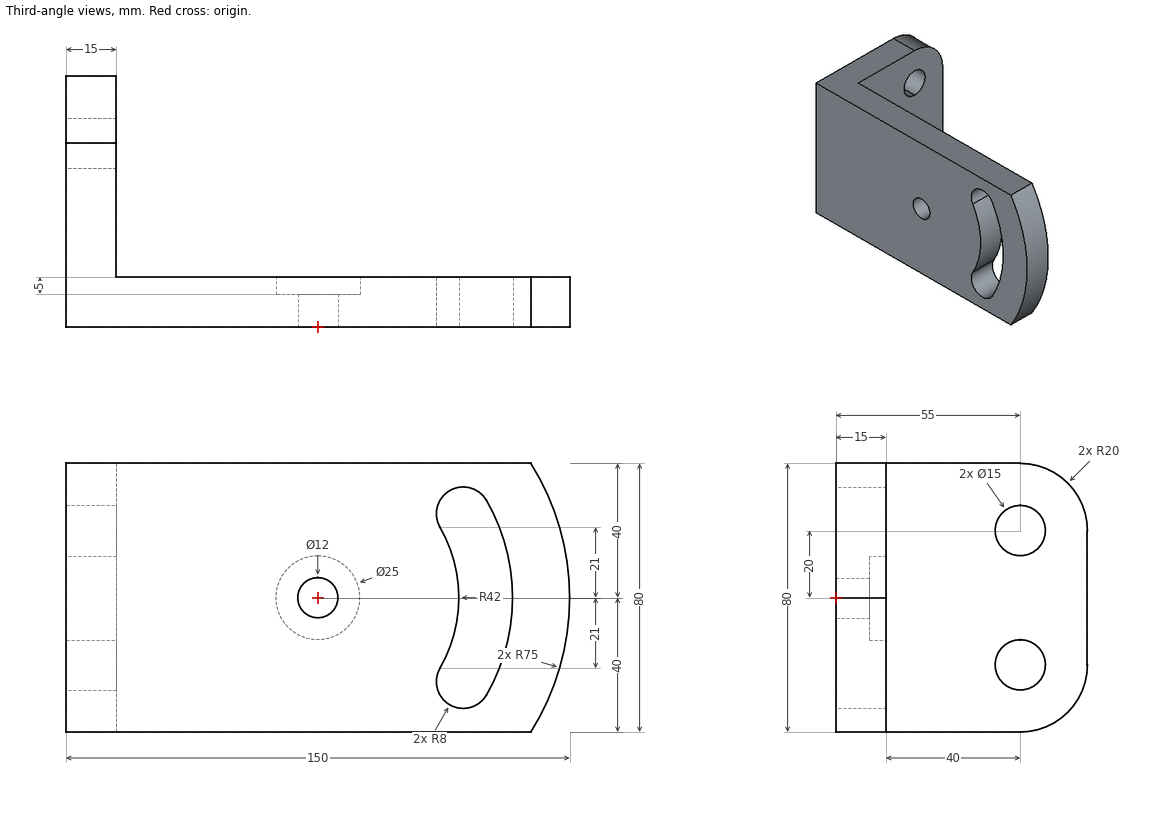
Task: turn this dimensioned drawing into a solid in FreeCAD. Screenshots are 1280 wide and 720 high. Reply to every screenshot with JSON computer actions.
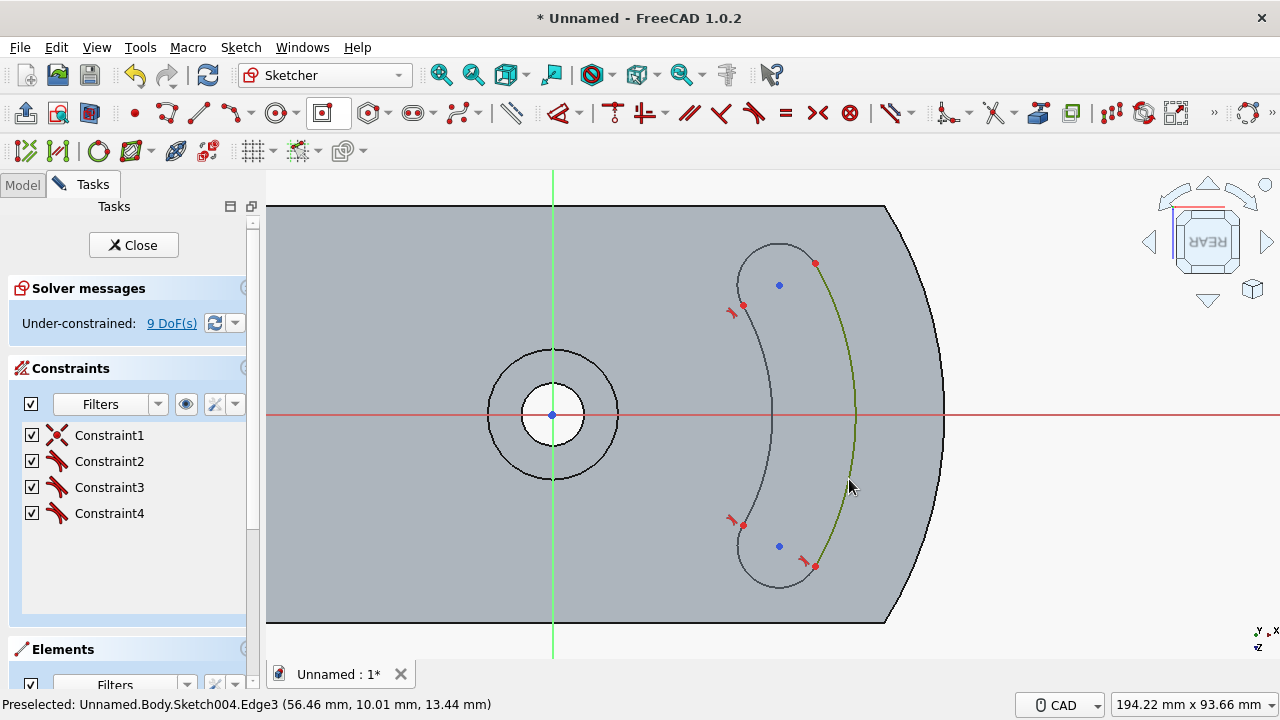
{"action": "left_click", "coordinate": [783, 244]}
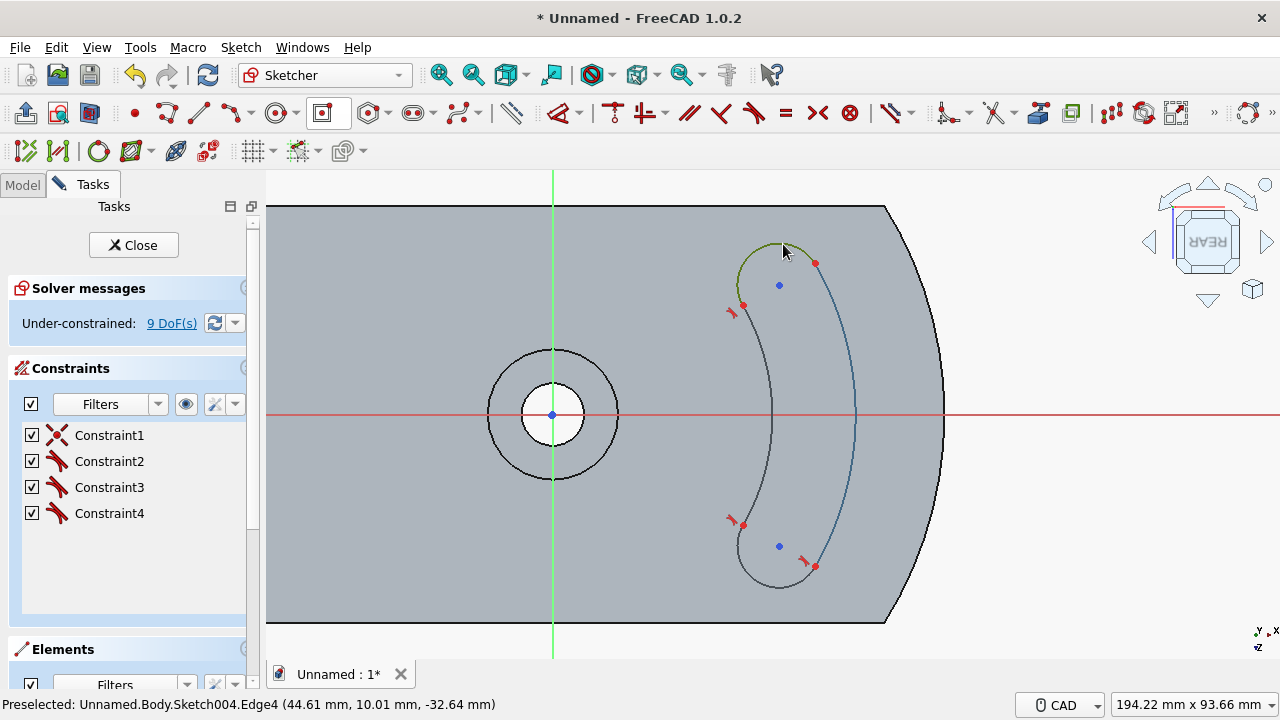
{"action": "left_click", "coordinate": [754, 114]}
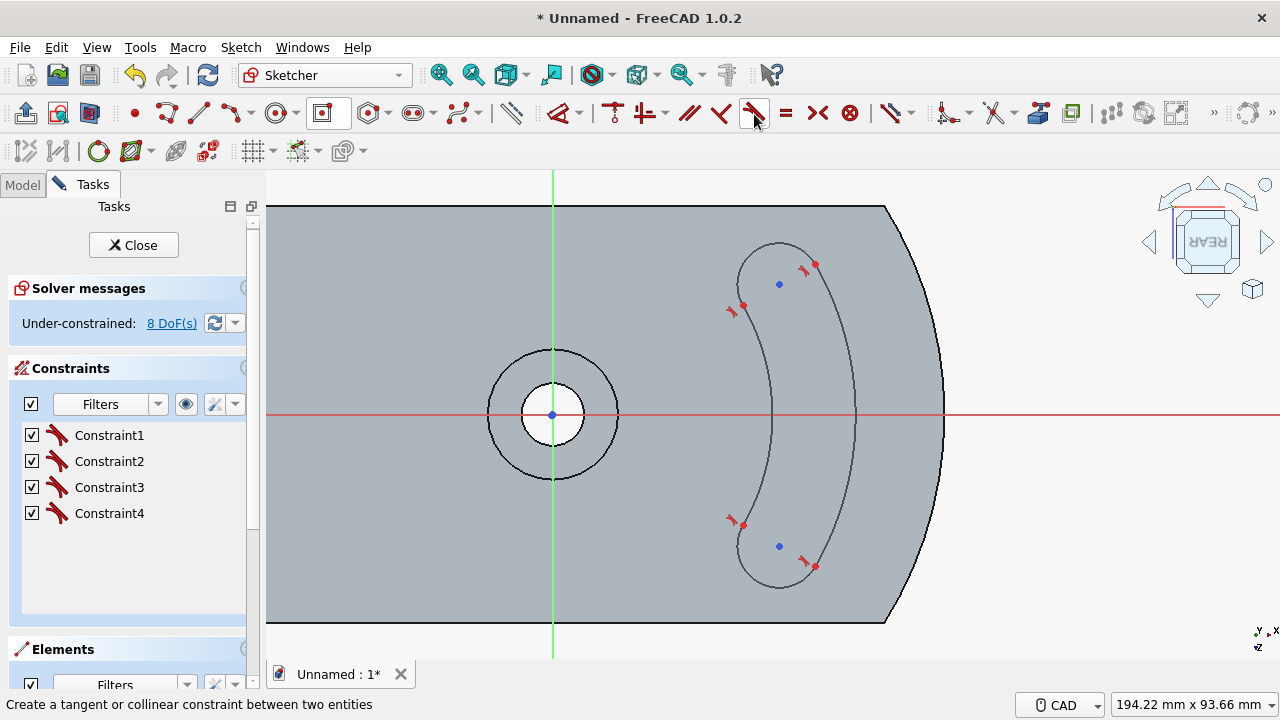
{"action": "left_click", "coordinate": [768, 461]}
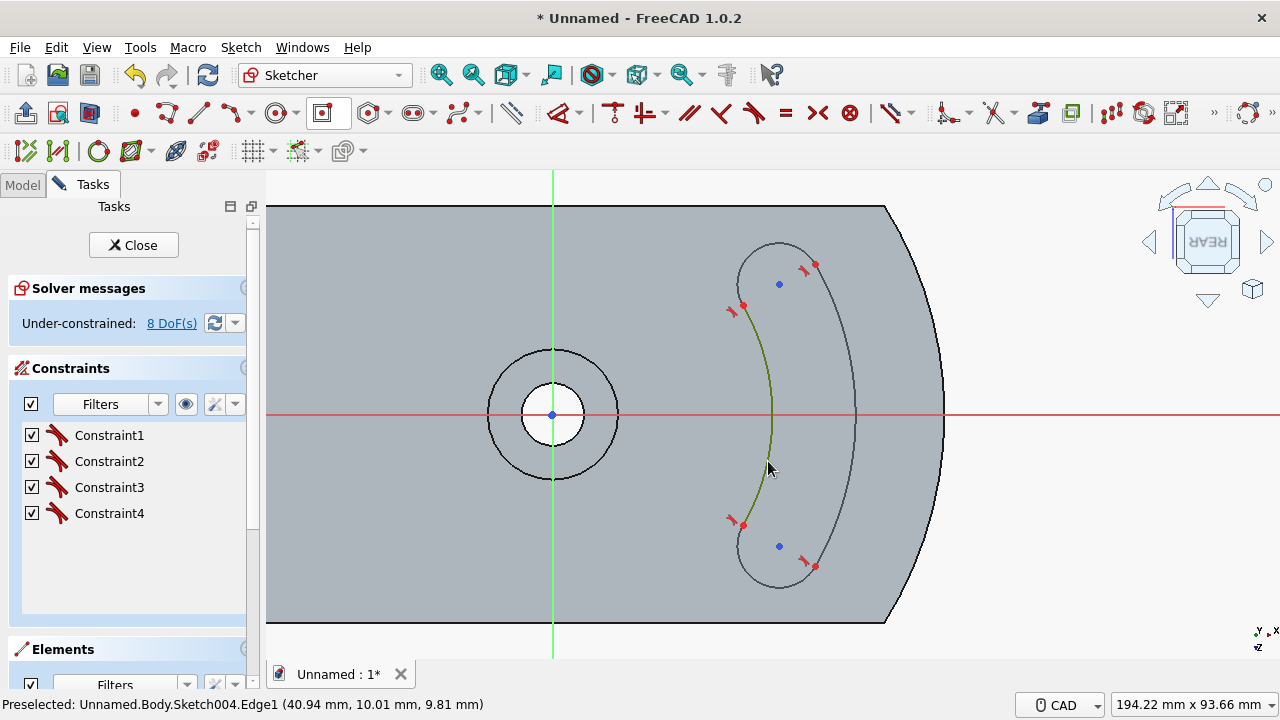
{"action": "left_click", "coordinate": [849, 479]}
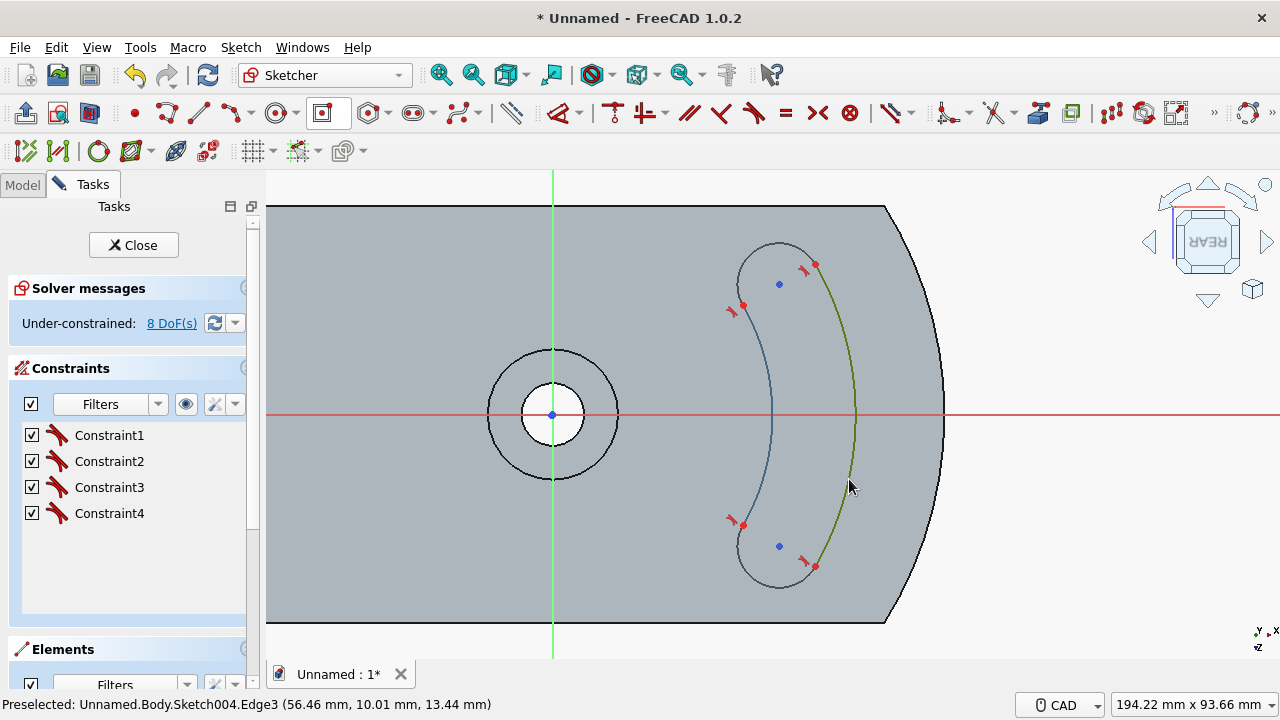
{"action": "left_click", "coordinate": [614, 114]}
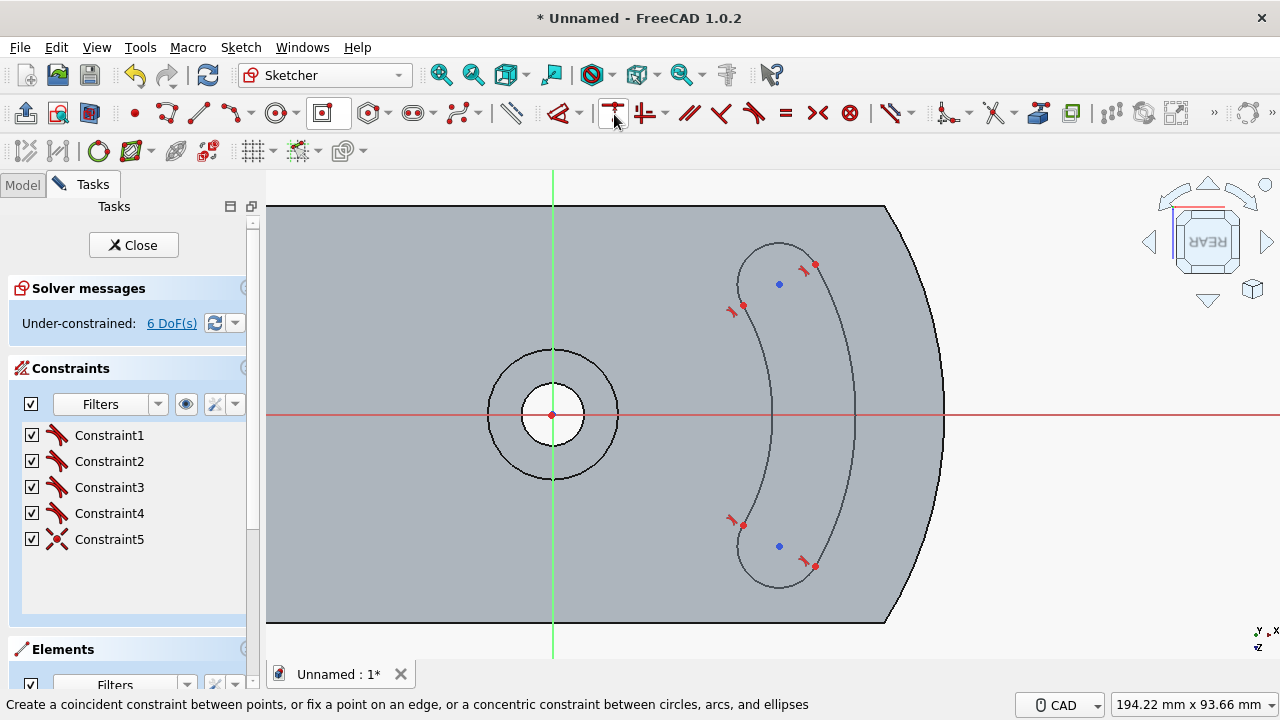
{"action": "left_click_drag", "start_coordinate": [542, 404], "coordinate": [563, 425]}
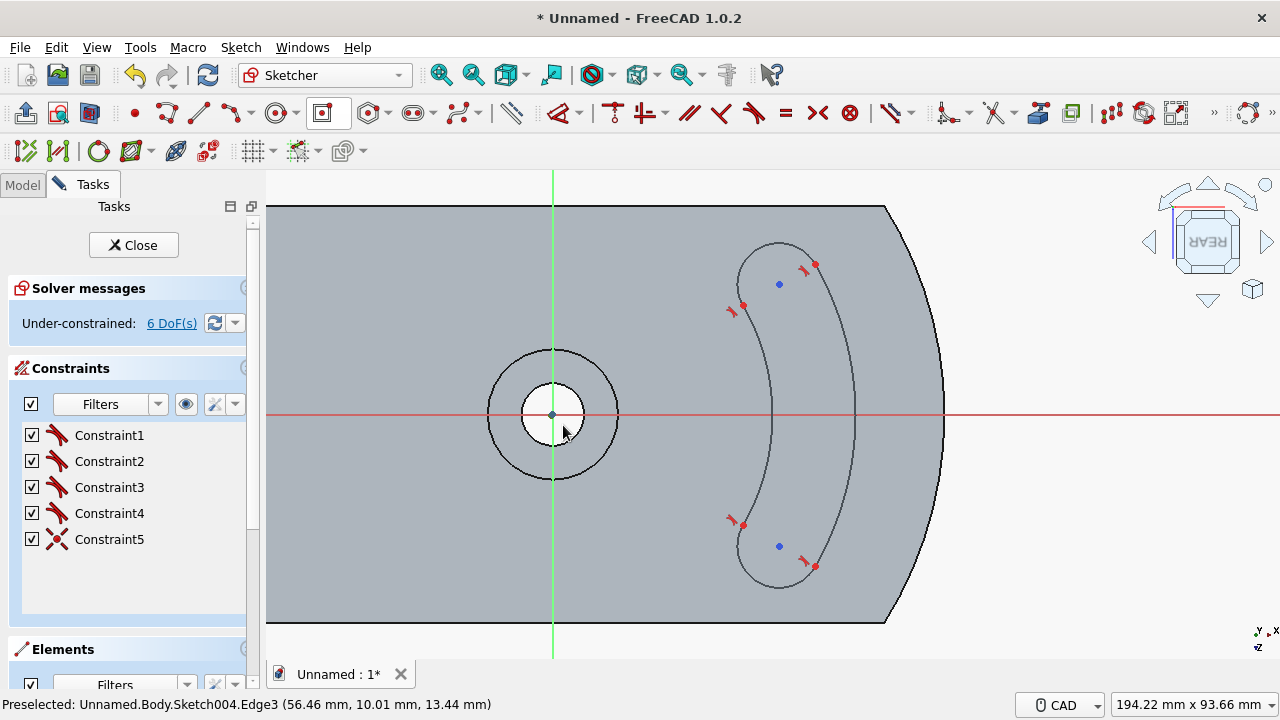
{"action": "left_click", "coordinate": [614, 114]}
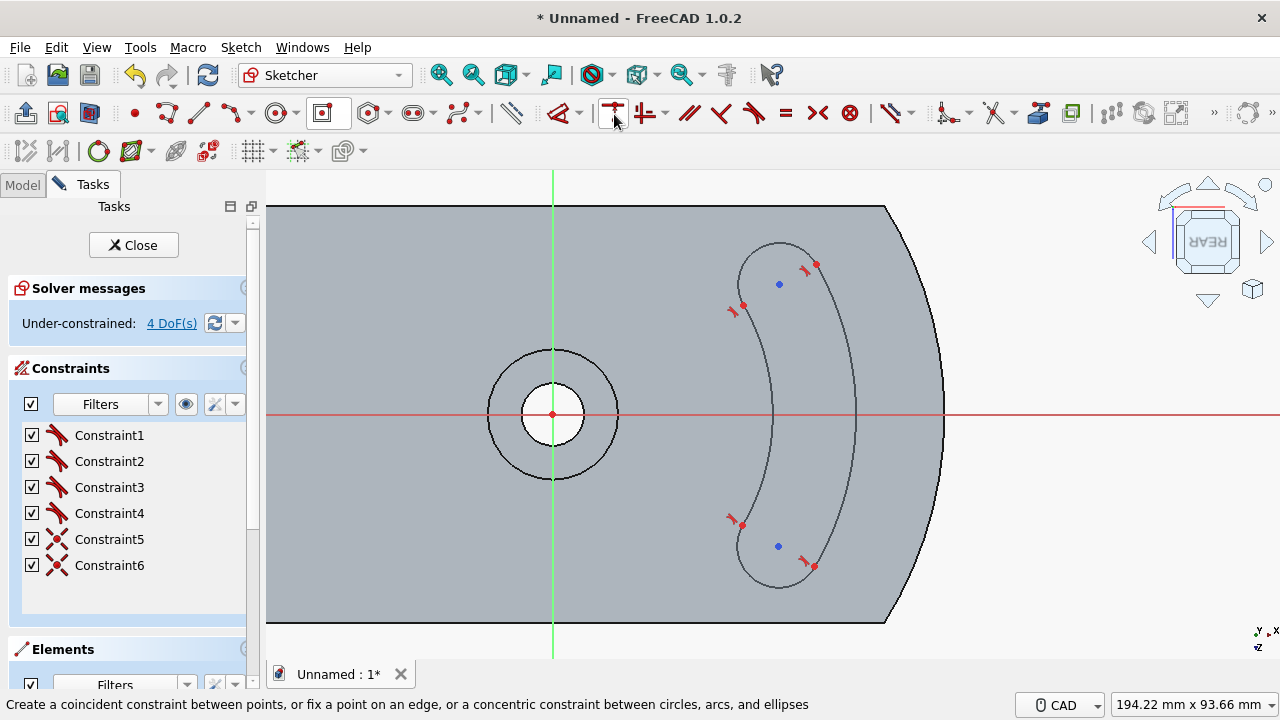
{"action": "left_click", "coordinate": [558, 114]}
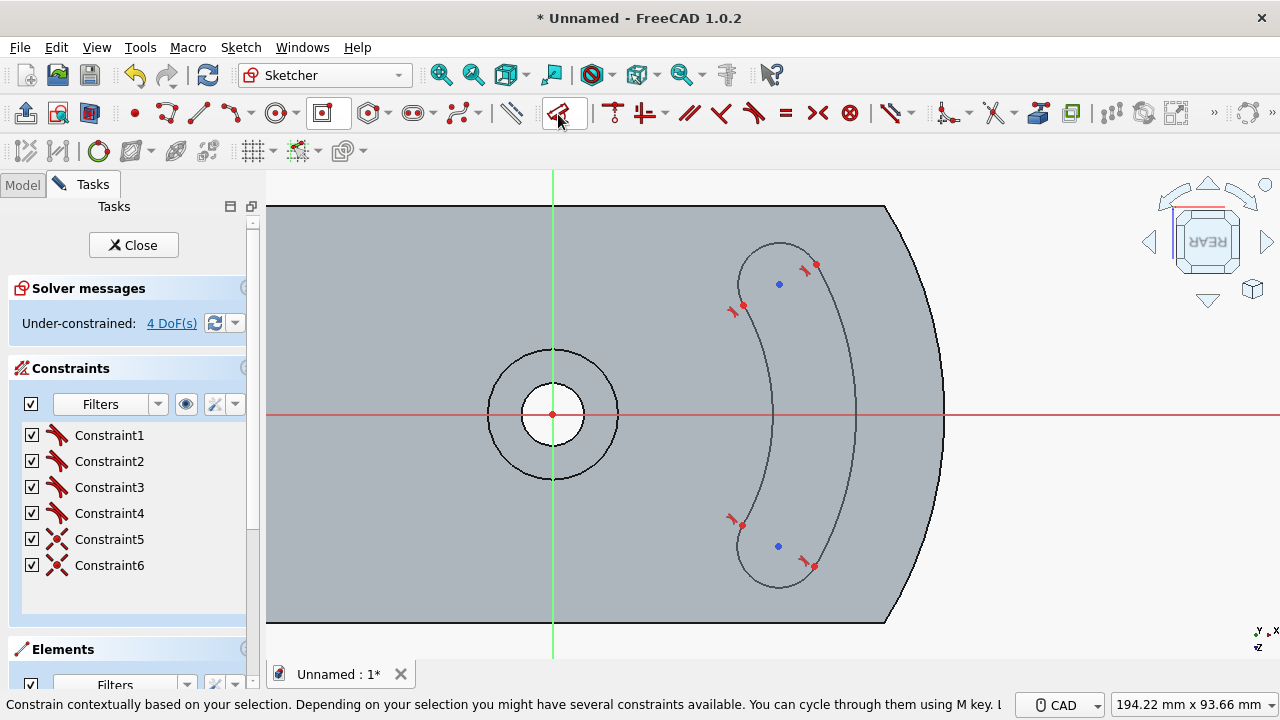
{"action": "left_click", "coordinate": [768, 461]}
{"action": "left_click", "coordinate": [799, 468]}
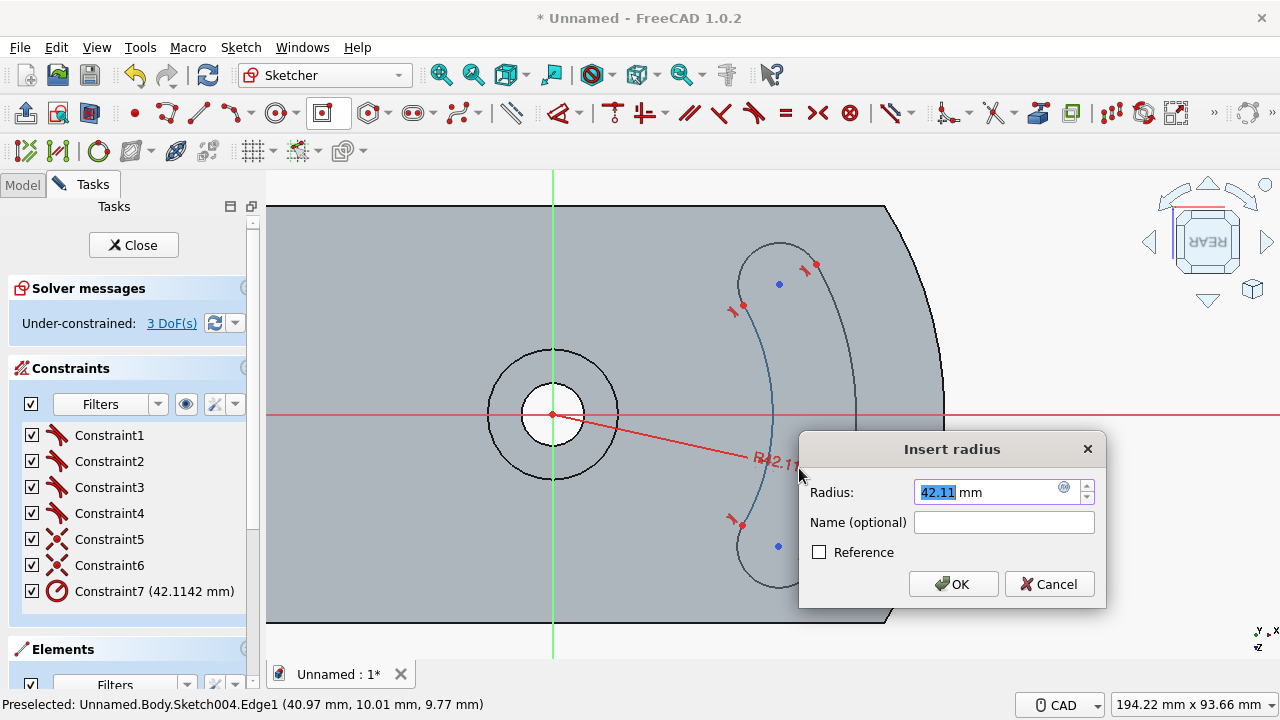
{"action": "type", "text": "42"}
{"action": "key", "text": "Return"}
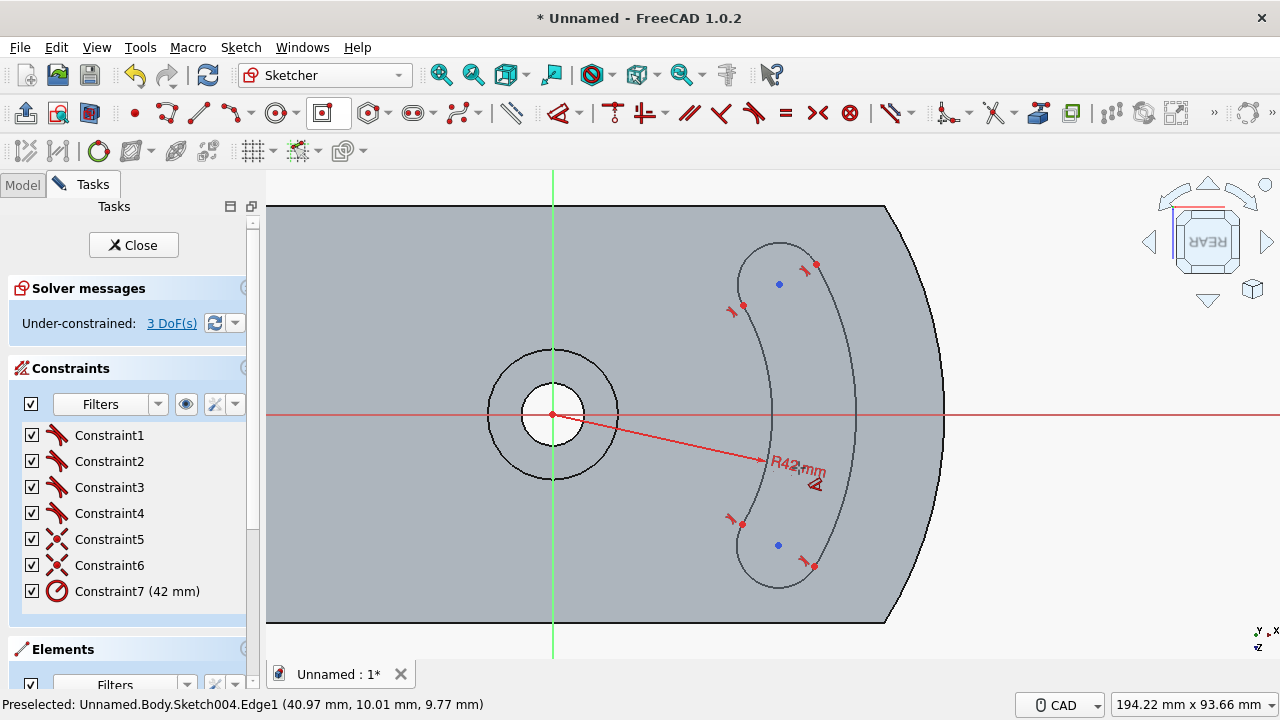
{"action": "left_click", "coordinate": [740, 563]}
{"action": "left_click", "coordinate": [711, 576]}